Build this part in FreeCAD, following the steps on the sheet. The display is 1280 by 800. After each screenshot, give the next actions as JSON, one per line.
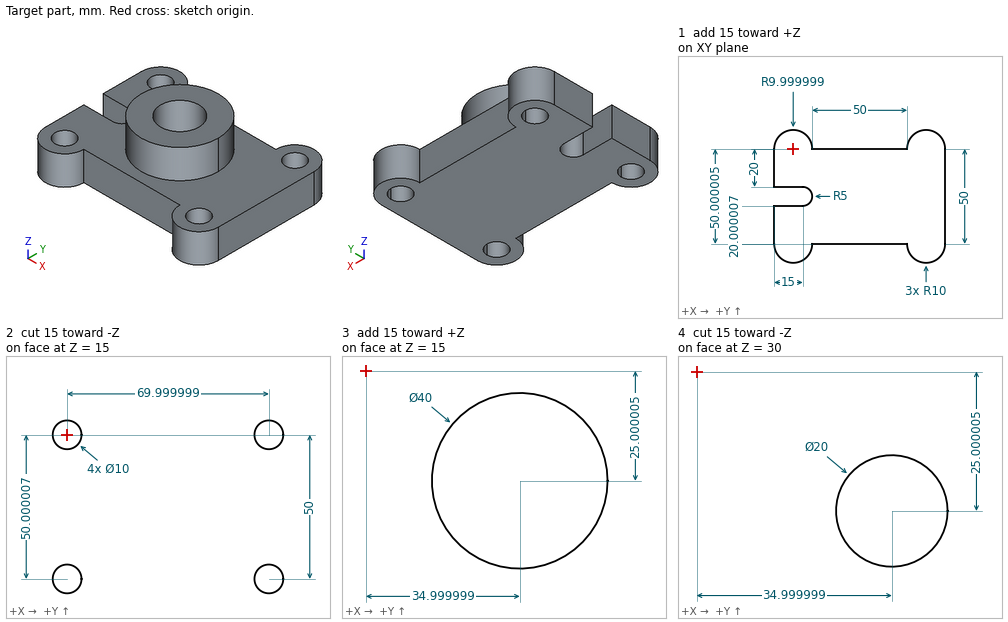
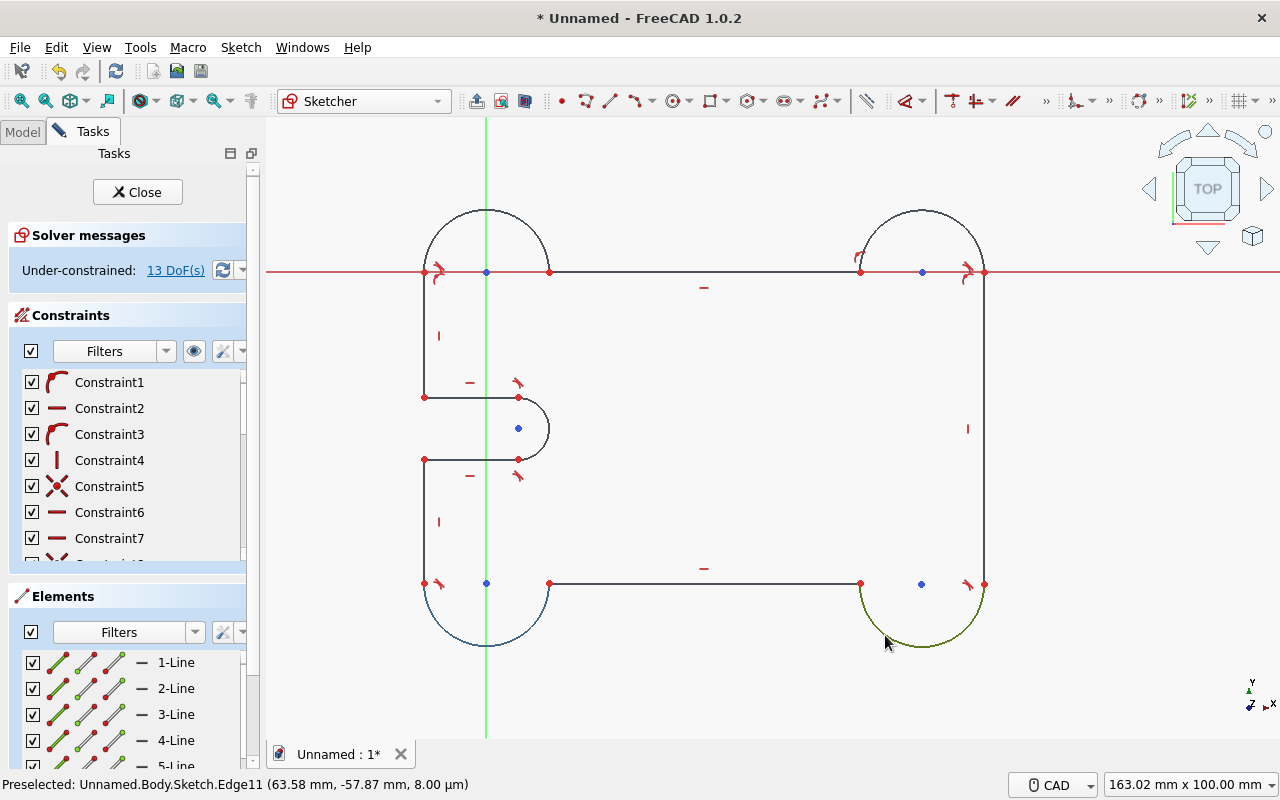
{"action": "left_click", "coordinate": [958, 222]}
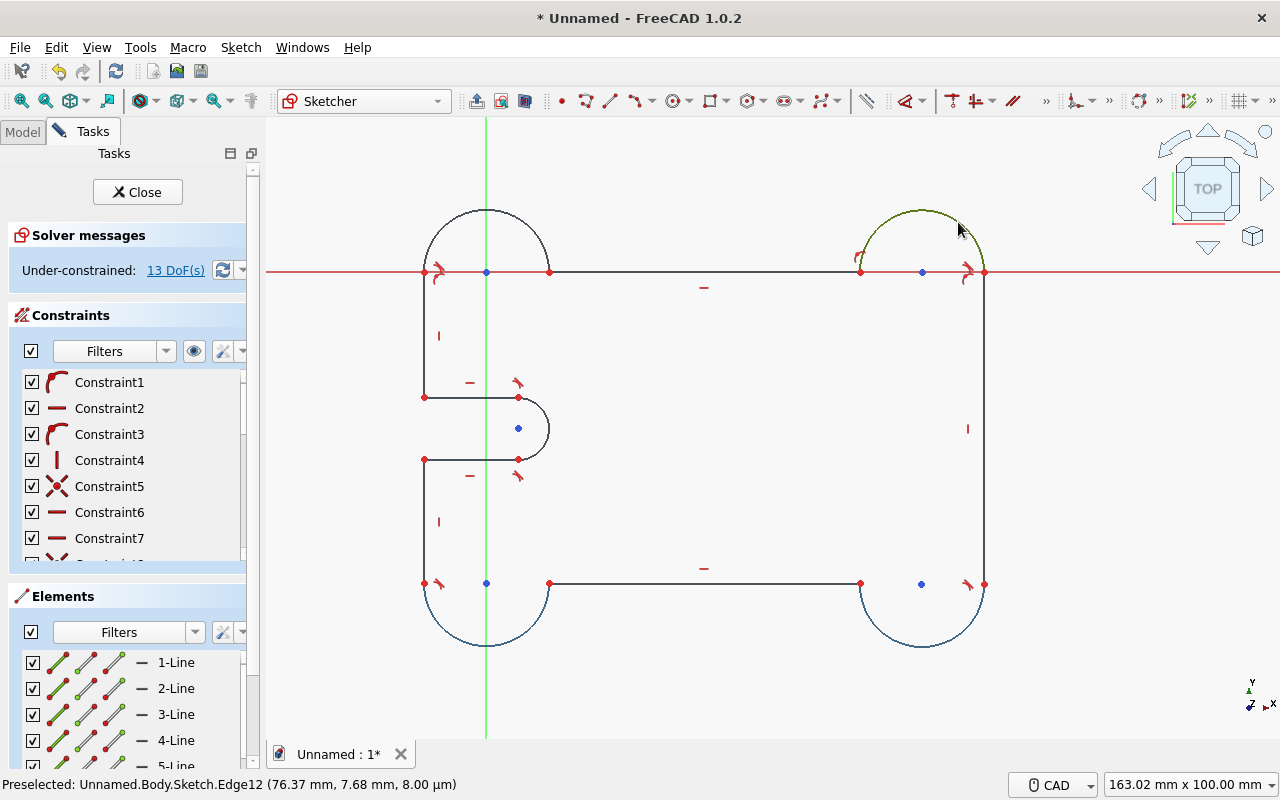
{"action": "key", "text": "e"}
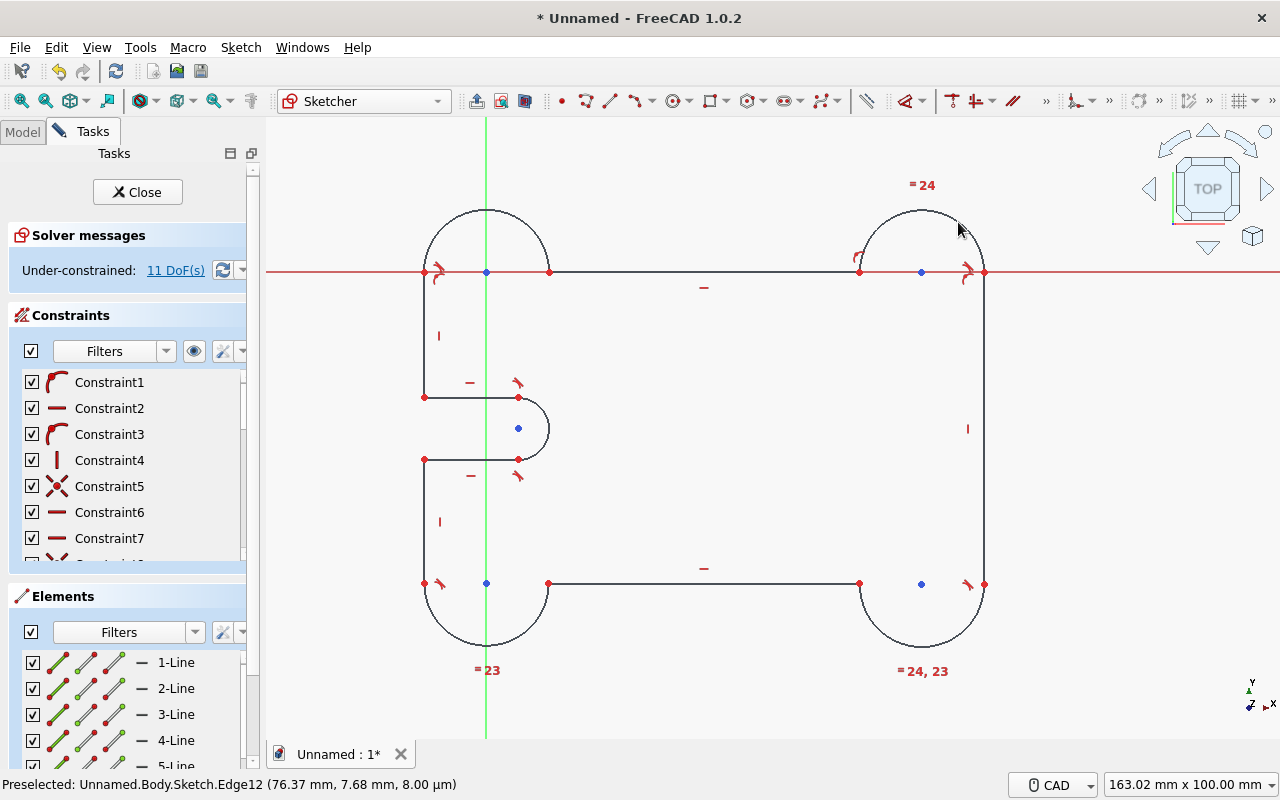
{"action": "left_click", "coordinate": [486, 272]}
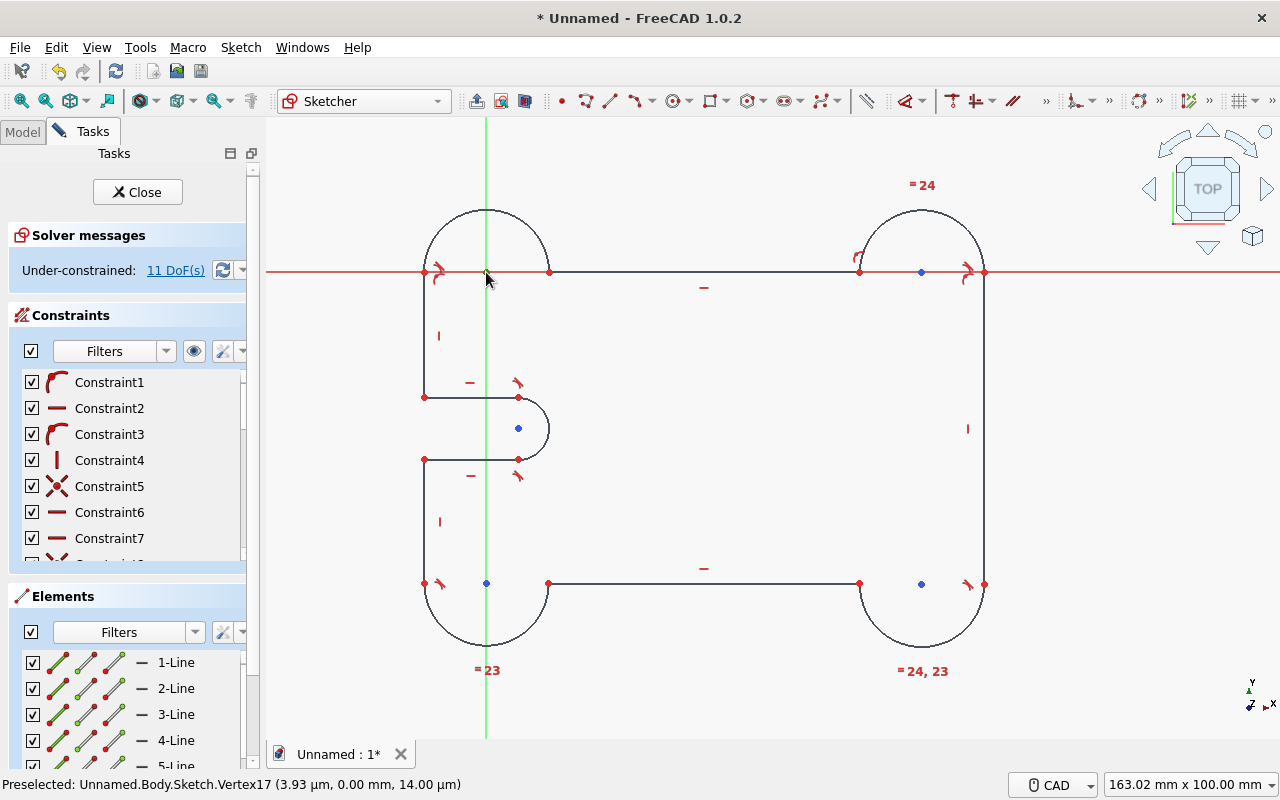
{"action": "left_click", "coordinate": [486, 590]}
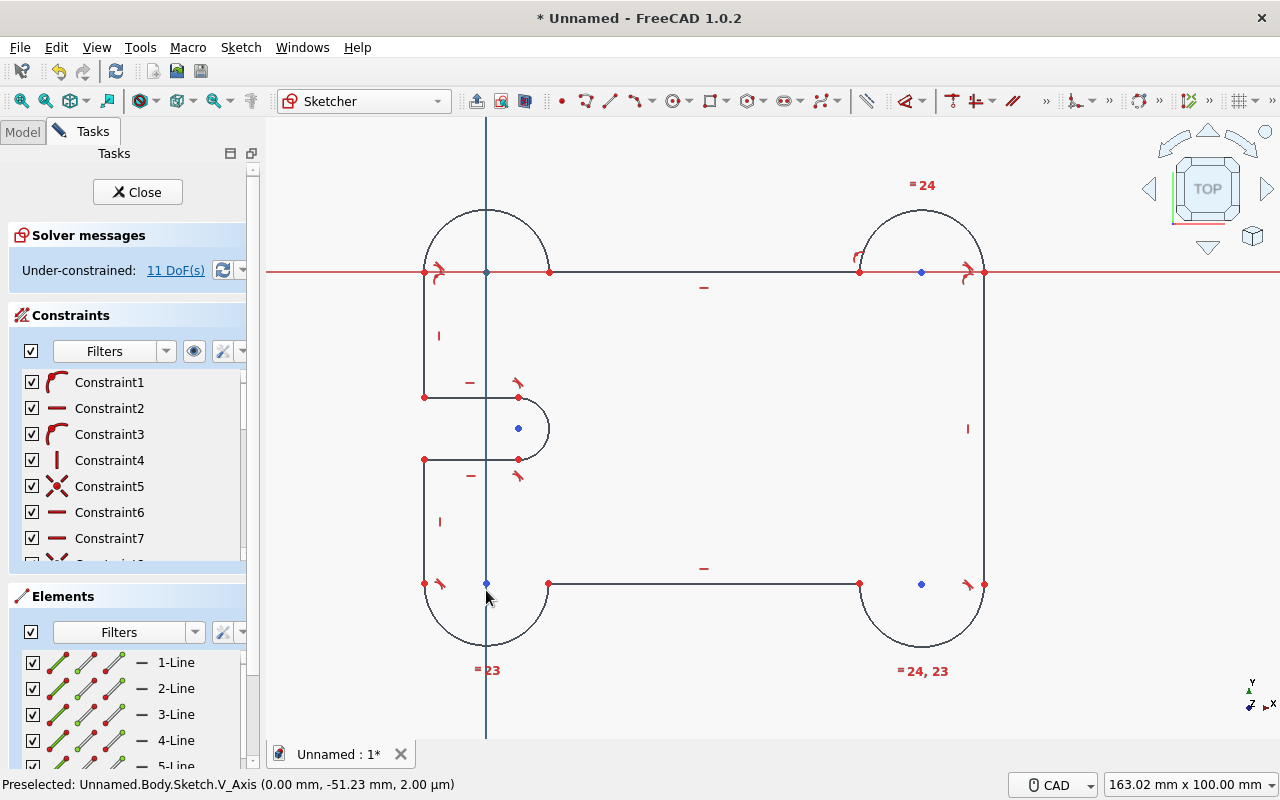
{"action": "left_click", "coordinate": [952, 102]}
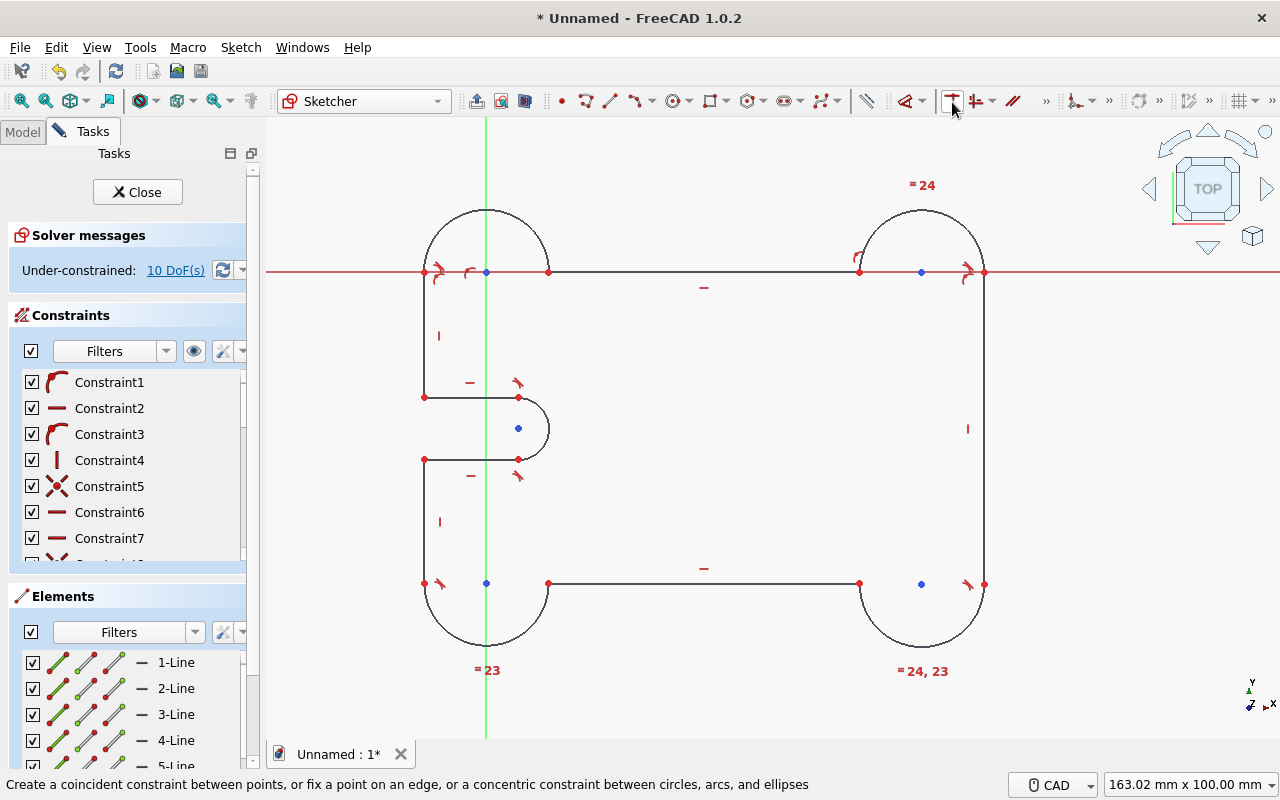
{"action": "left_click", "coordinate": [487, 584]}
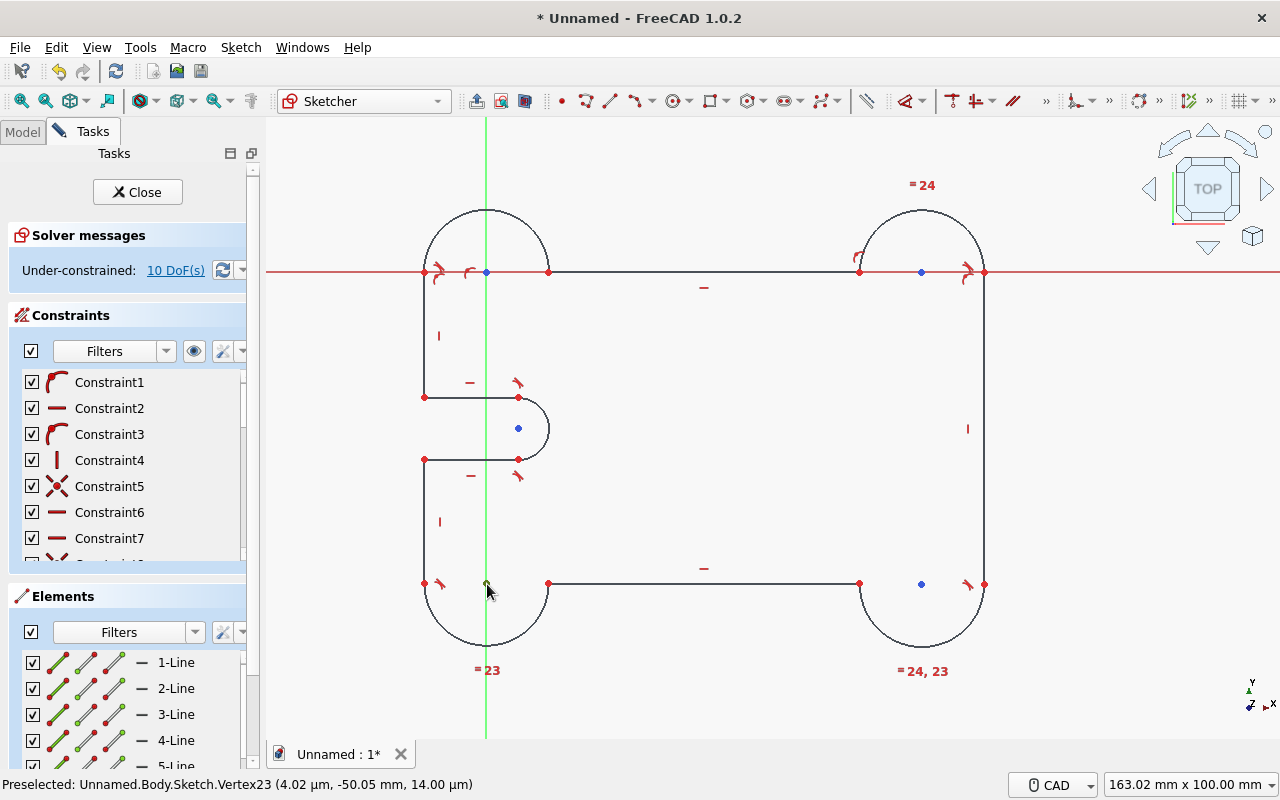
{"action": "left_click", "coordinate": [486, 590]}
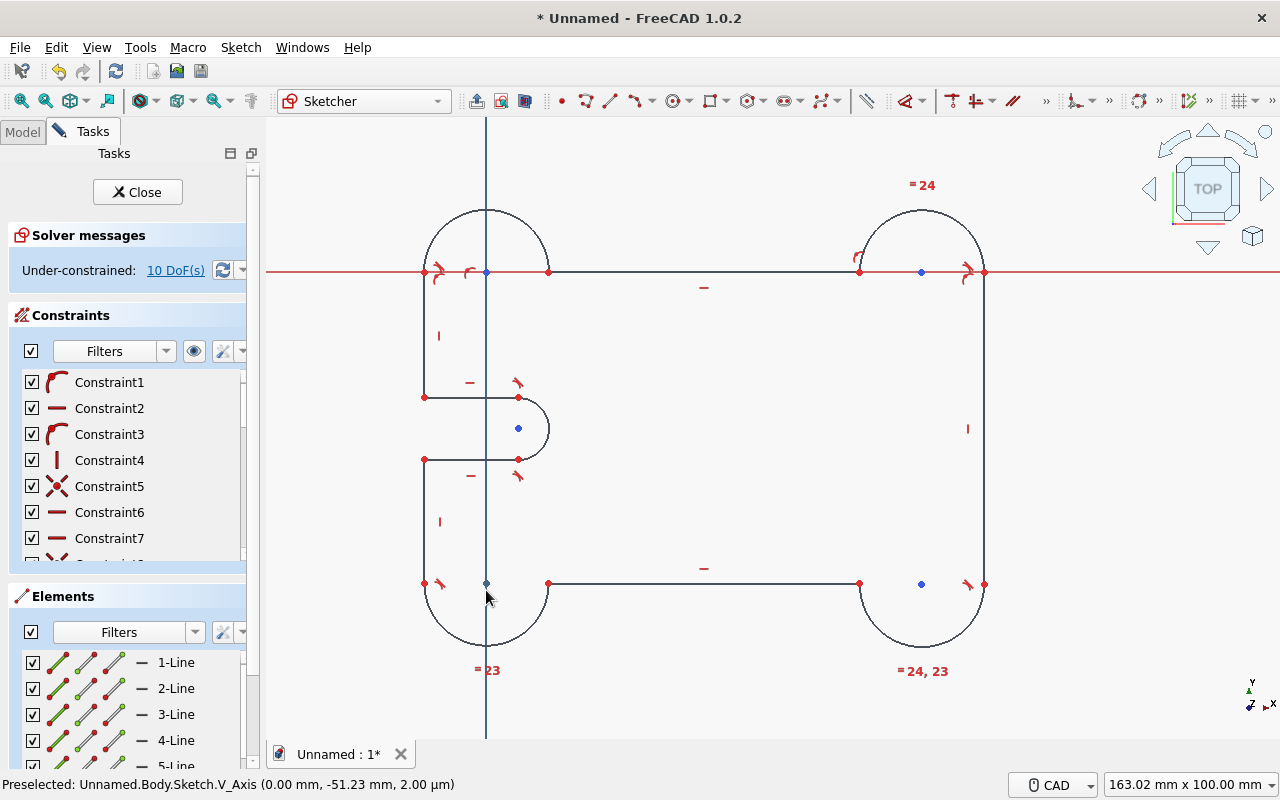
{"action": "left_click", "coordinate": [952, 102]}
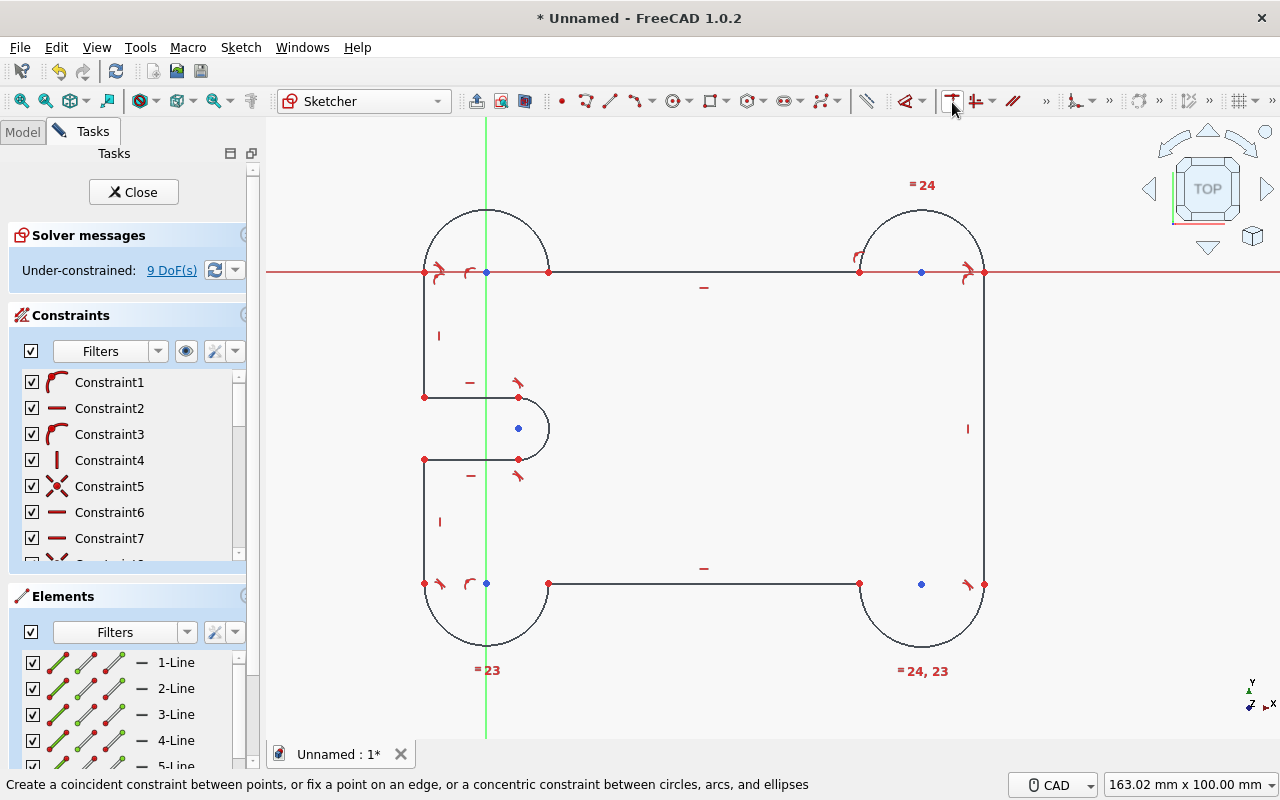
{"action": "left_click", "coordinate": [906, 102]}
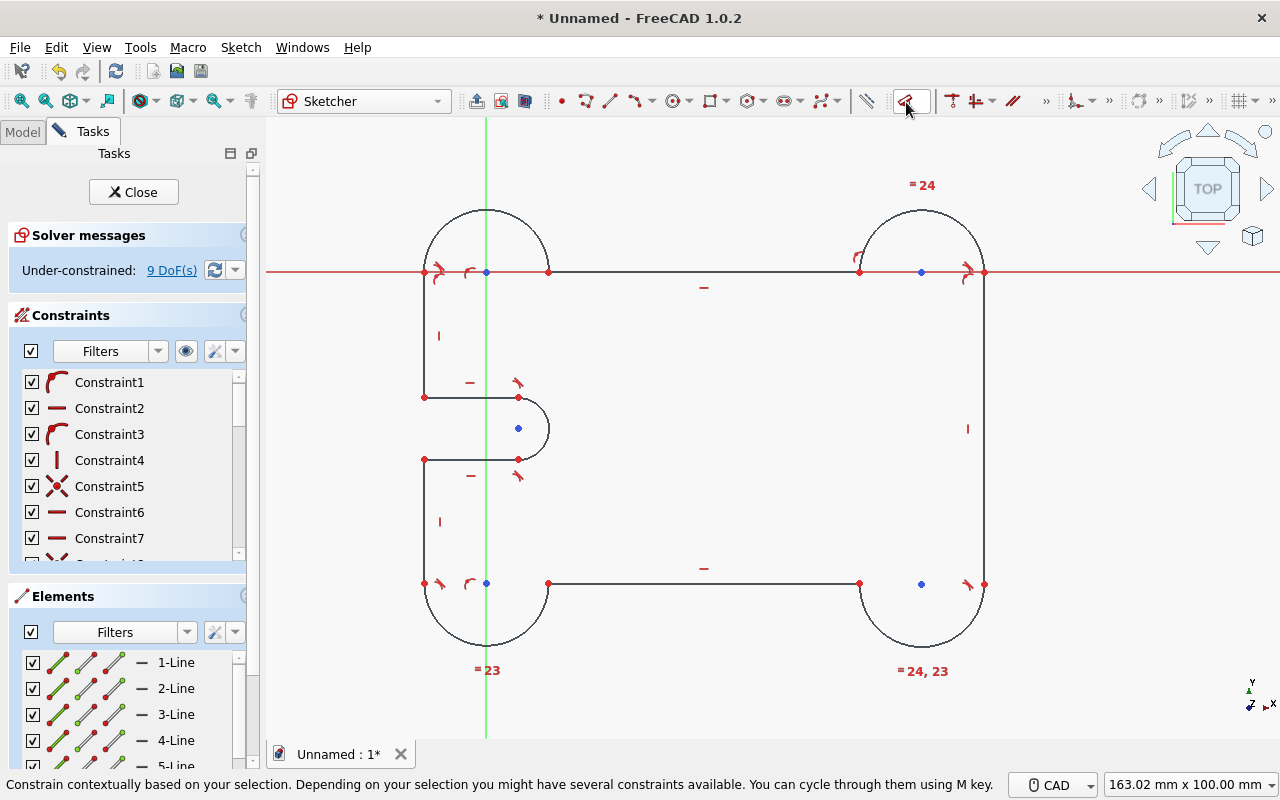
{"action": "left_click", "coordinate": [523, 222]}
{"action": "left_click", "coordinate": [542, 196]}